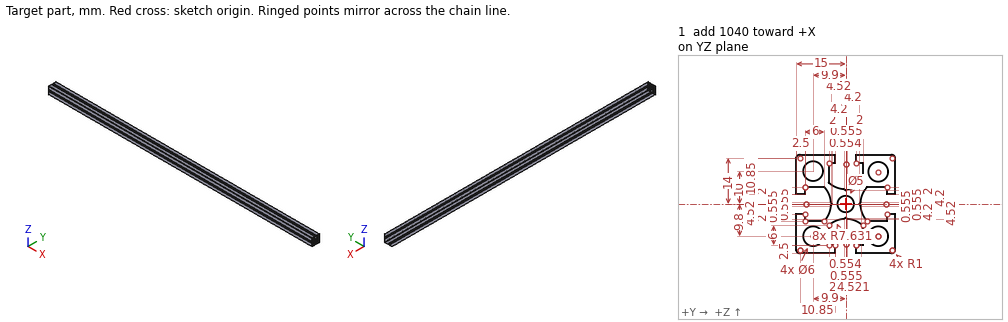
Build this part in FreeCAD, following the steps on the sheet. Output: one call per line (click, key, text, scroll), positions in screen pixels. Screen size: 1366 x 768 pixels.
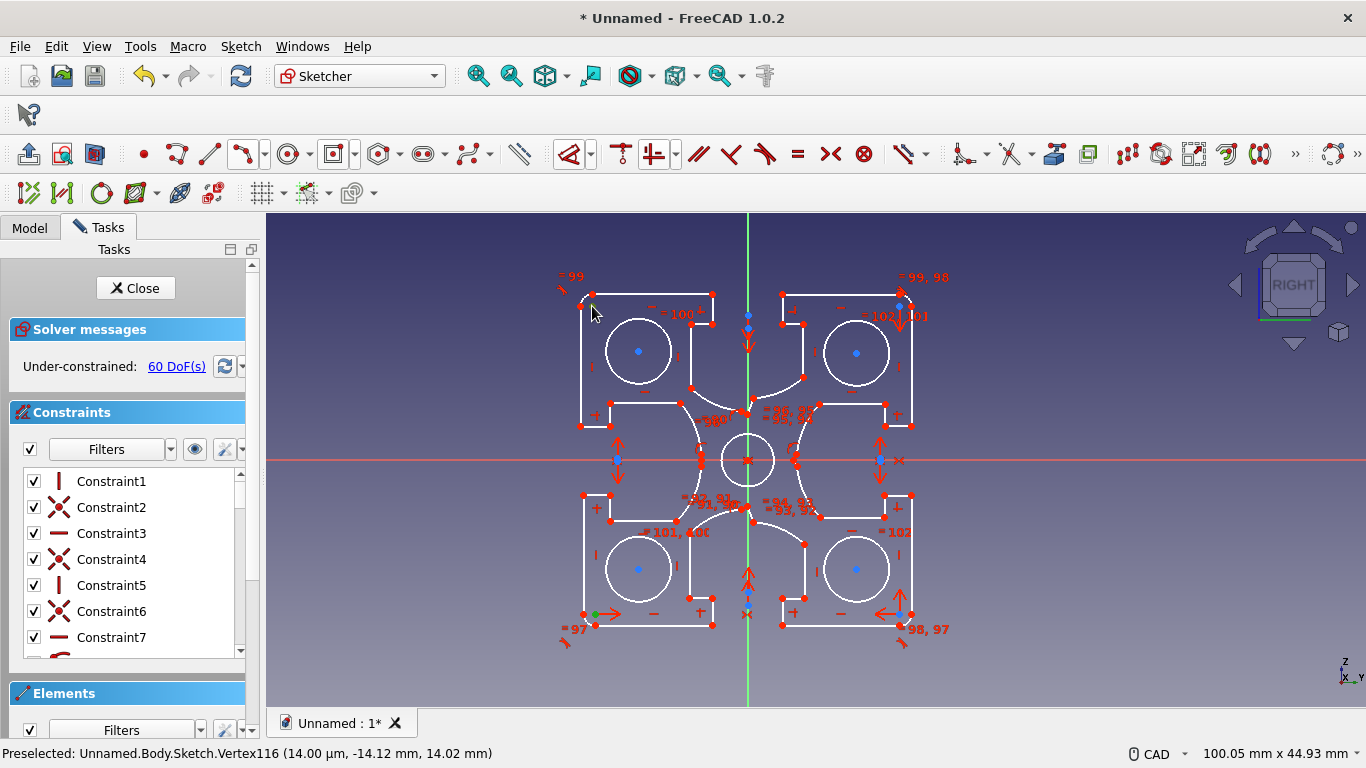
click(359, 460)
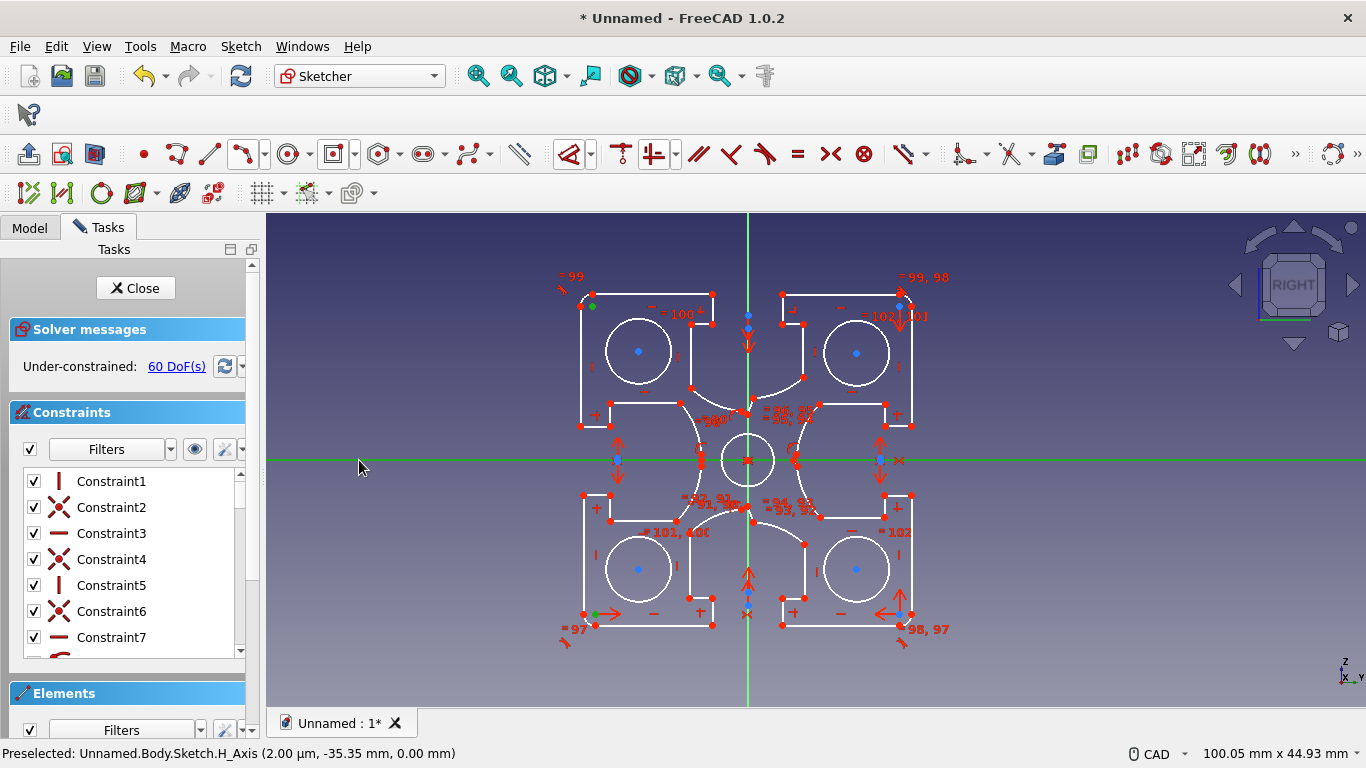
key(s)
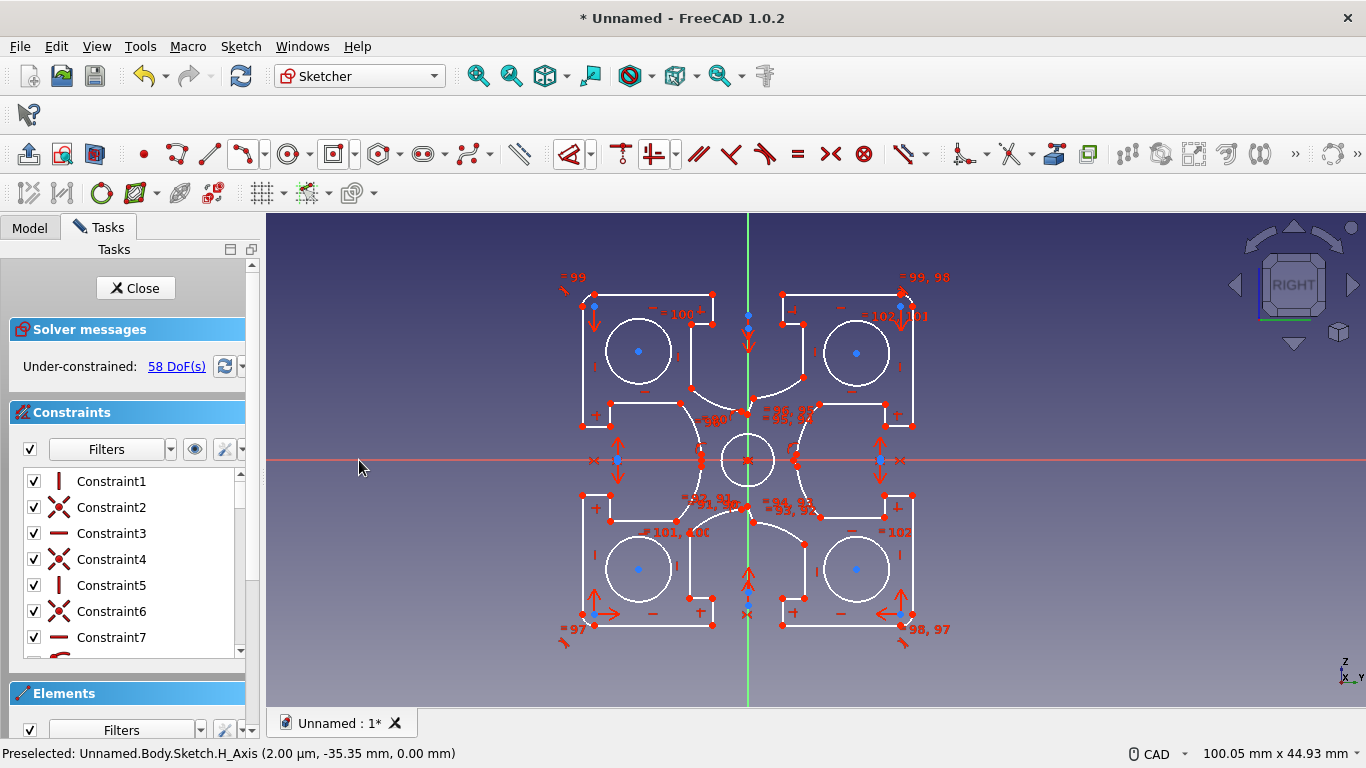
click(639, 569)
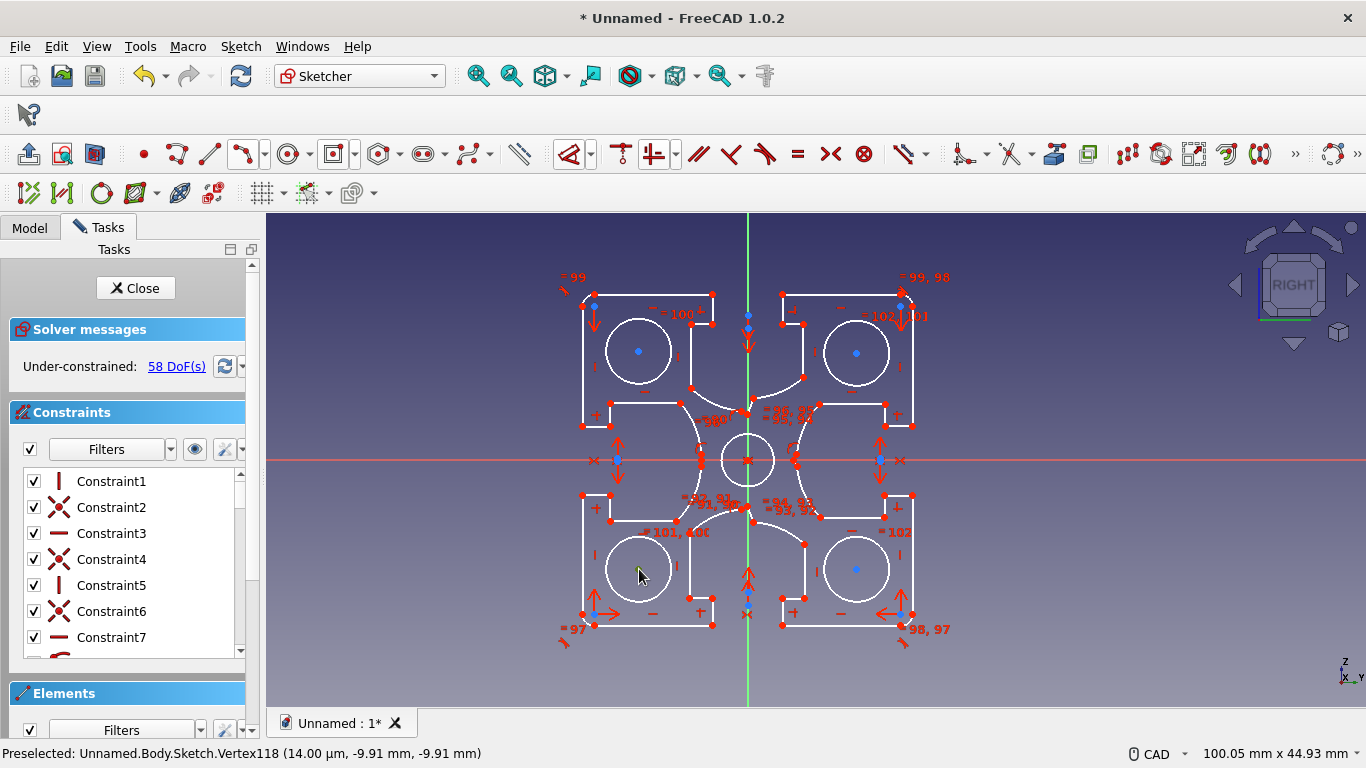
click(857, 569)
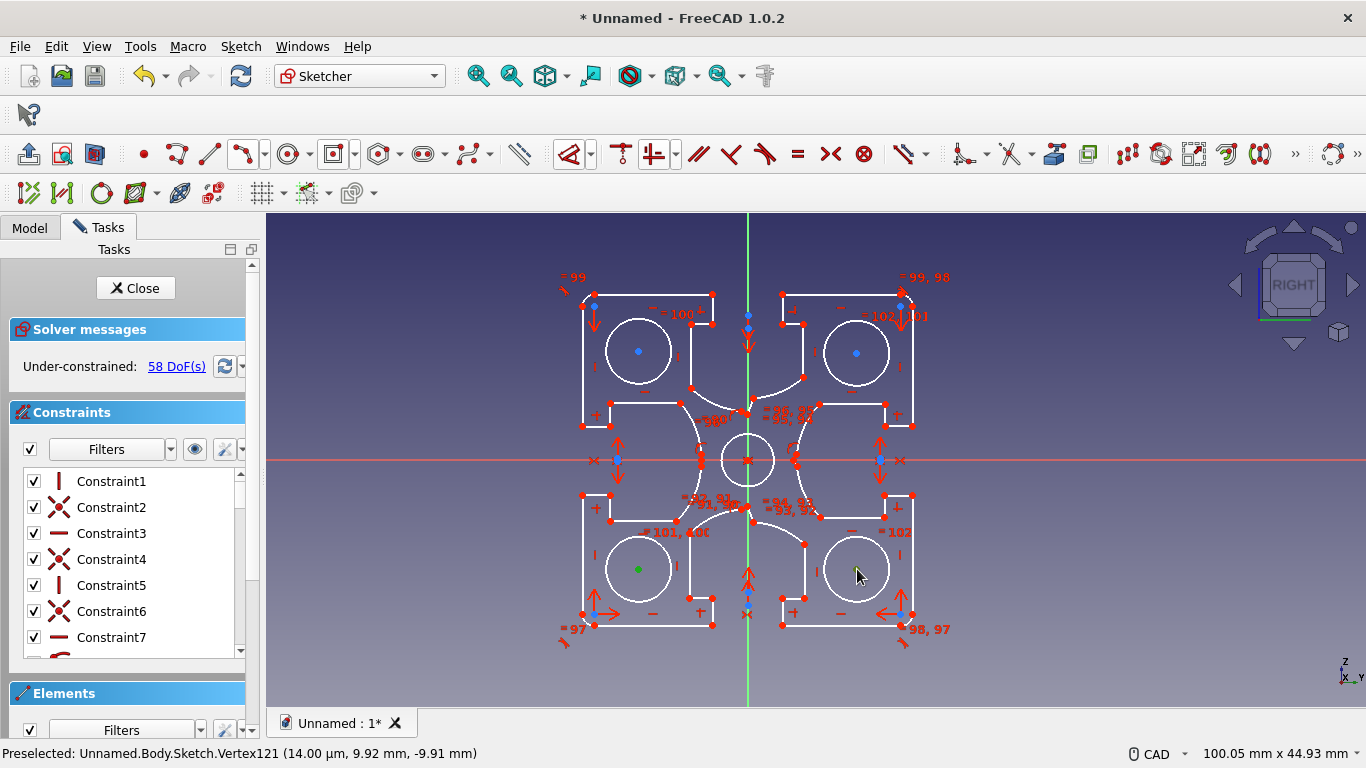
click(748, 648)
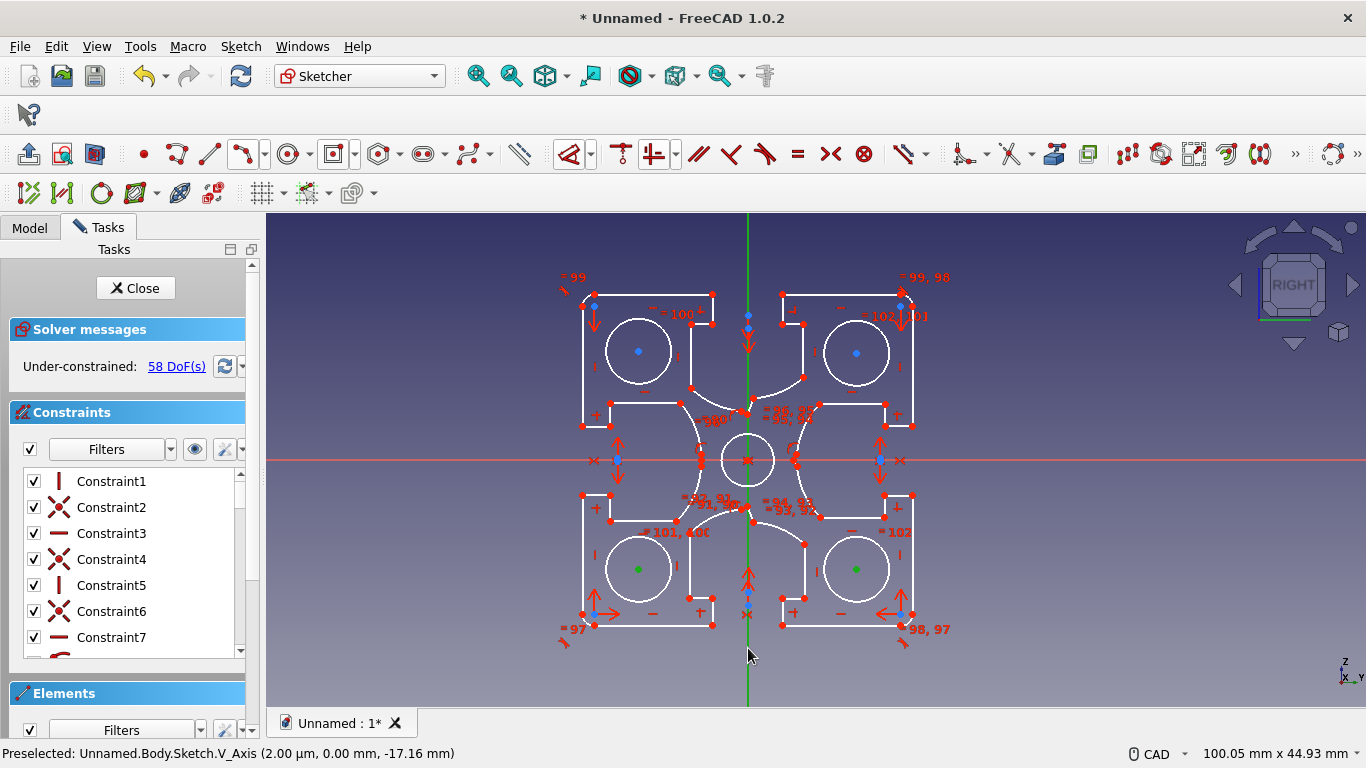
key(s)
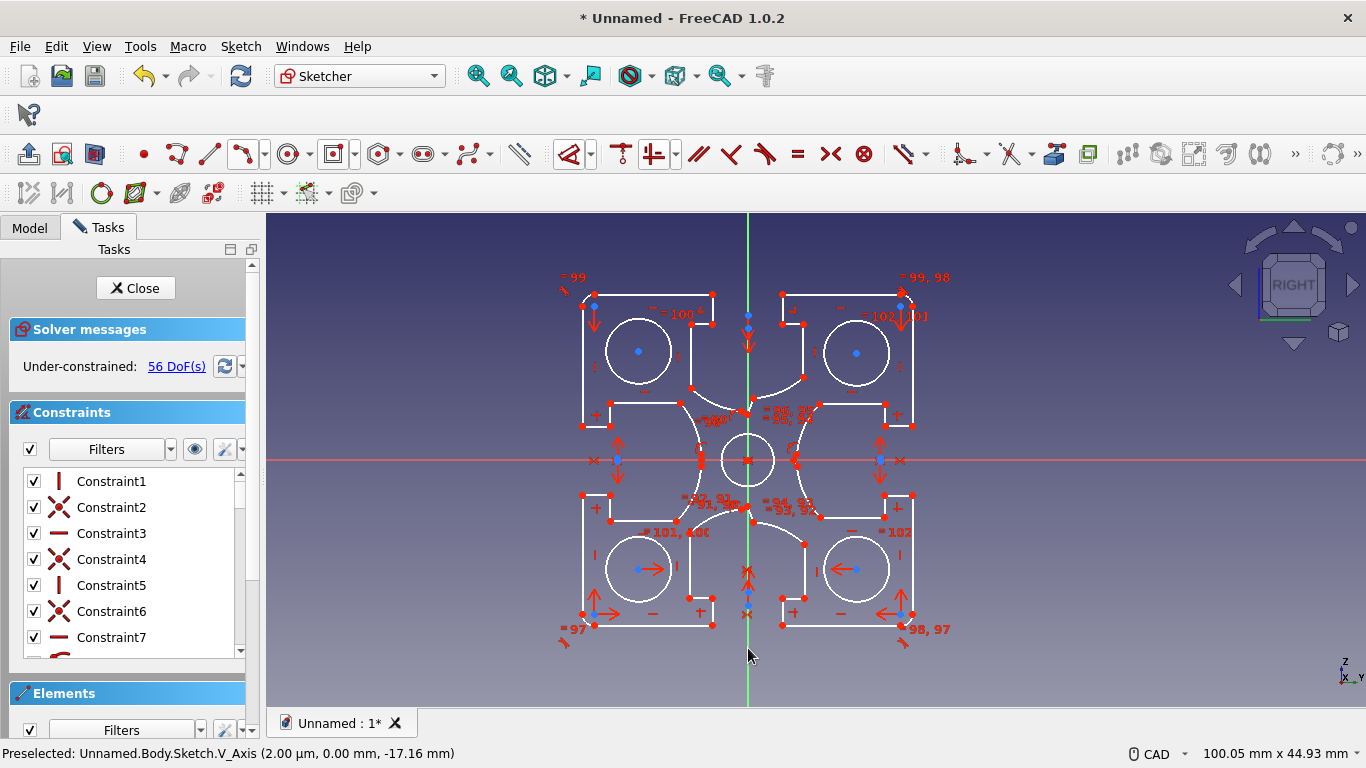
click(857, 353)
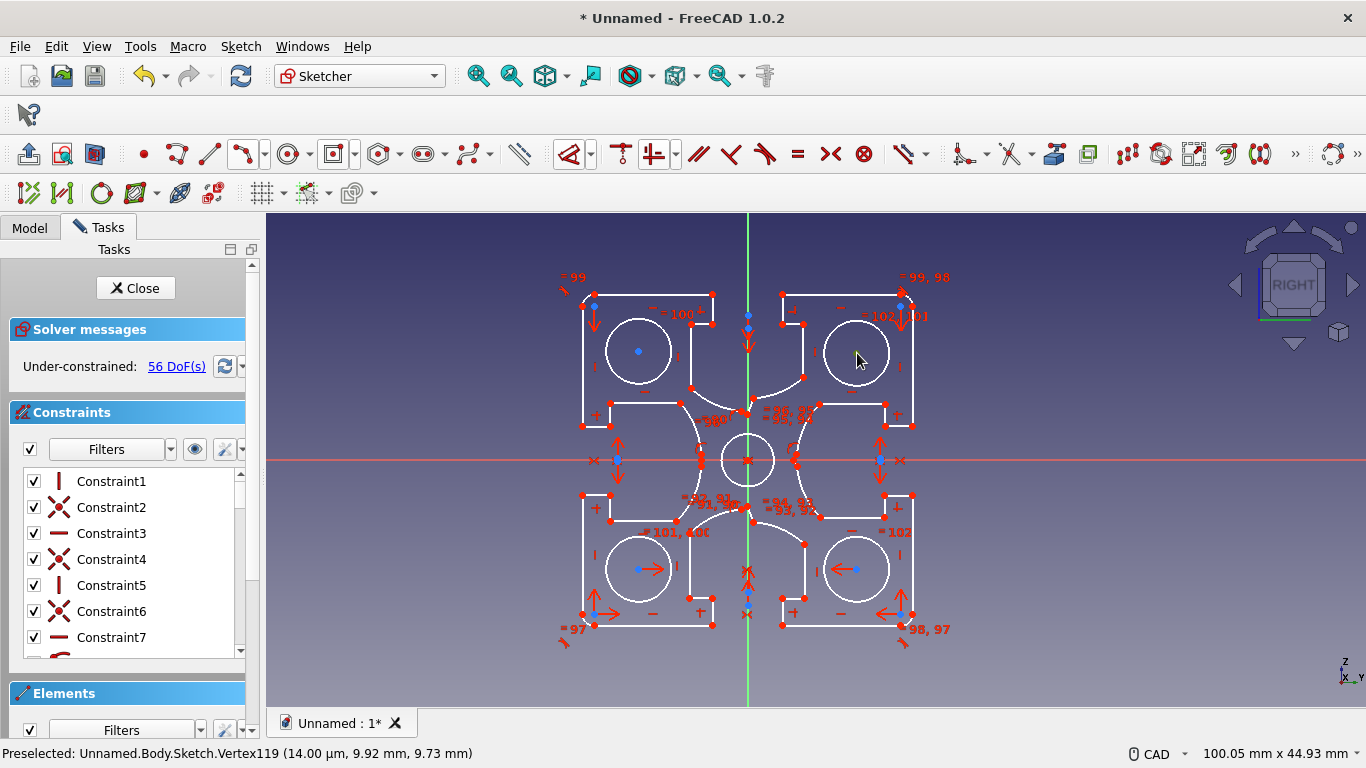
click(857, 569)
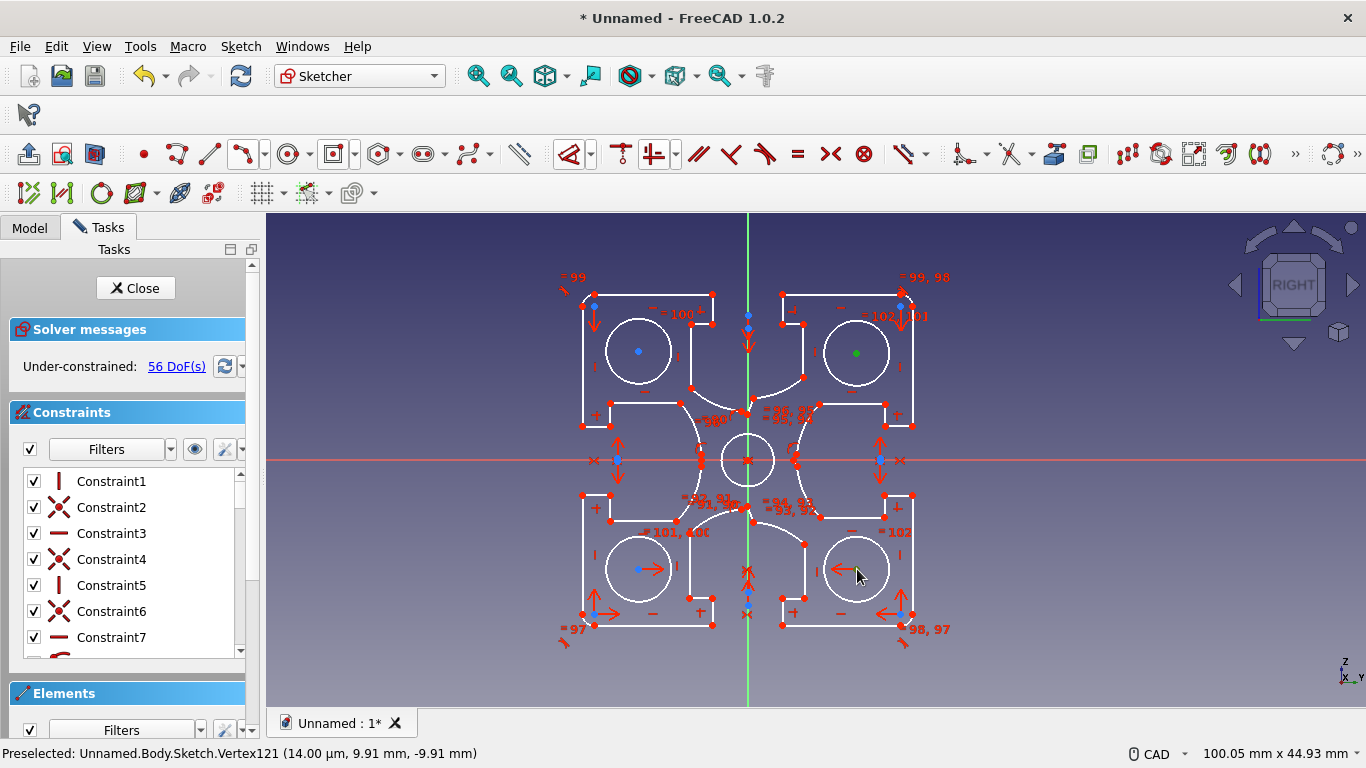
click(359, 460)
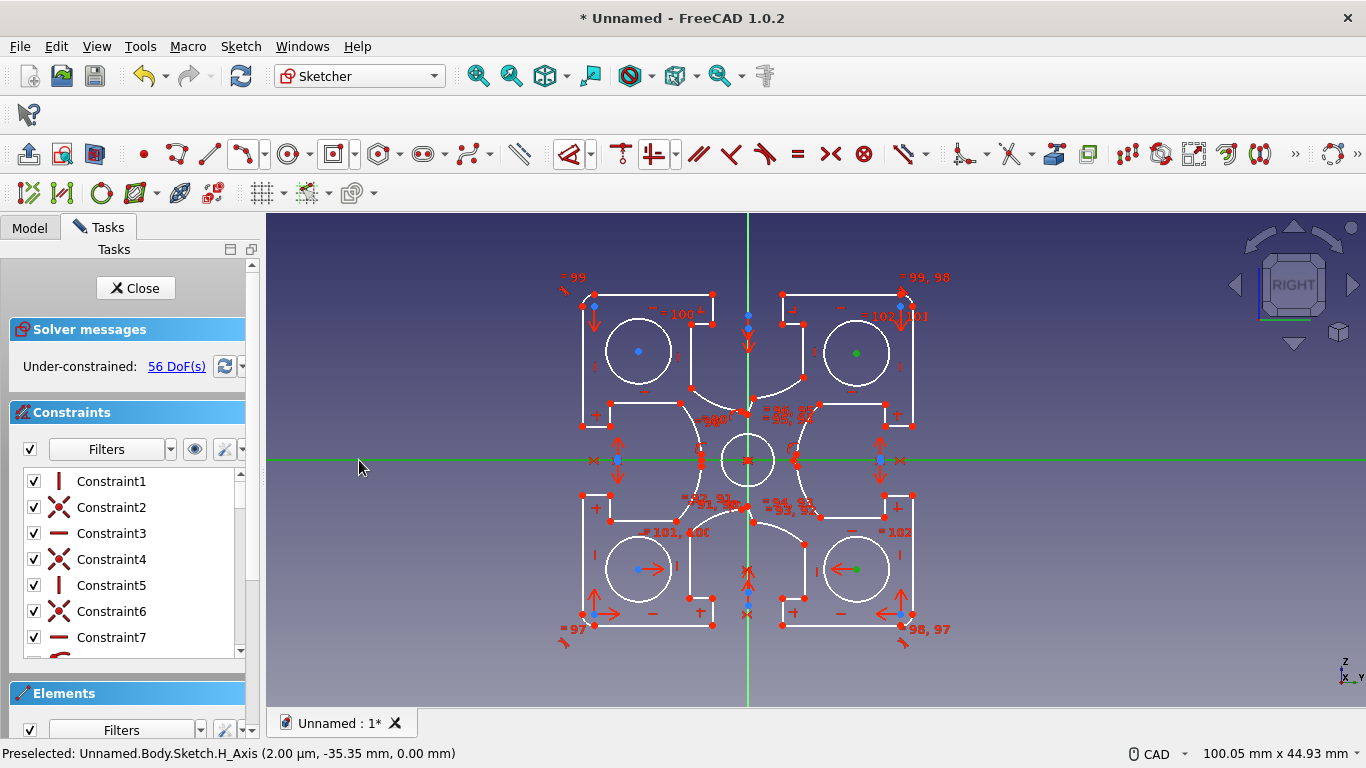
click(831, 154)